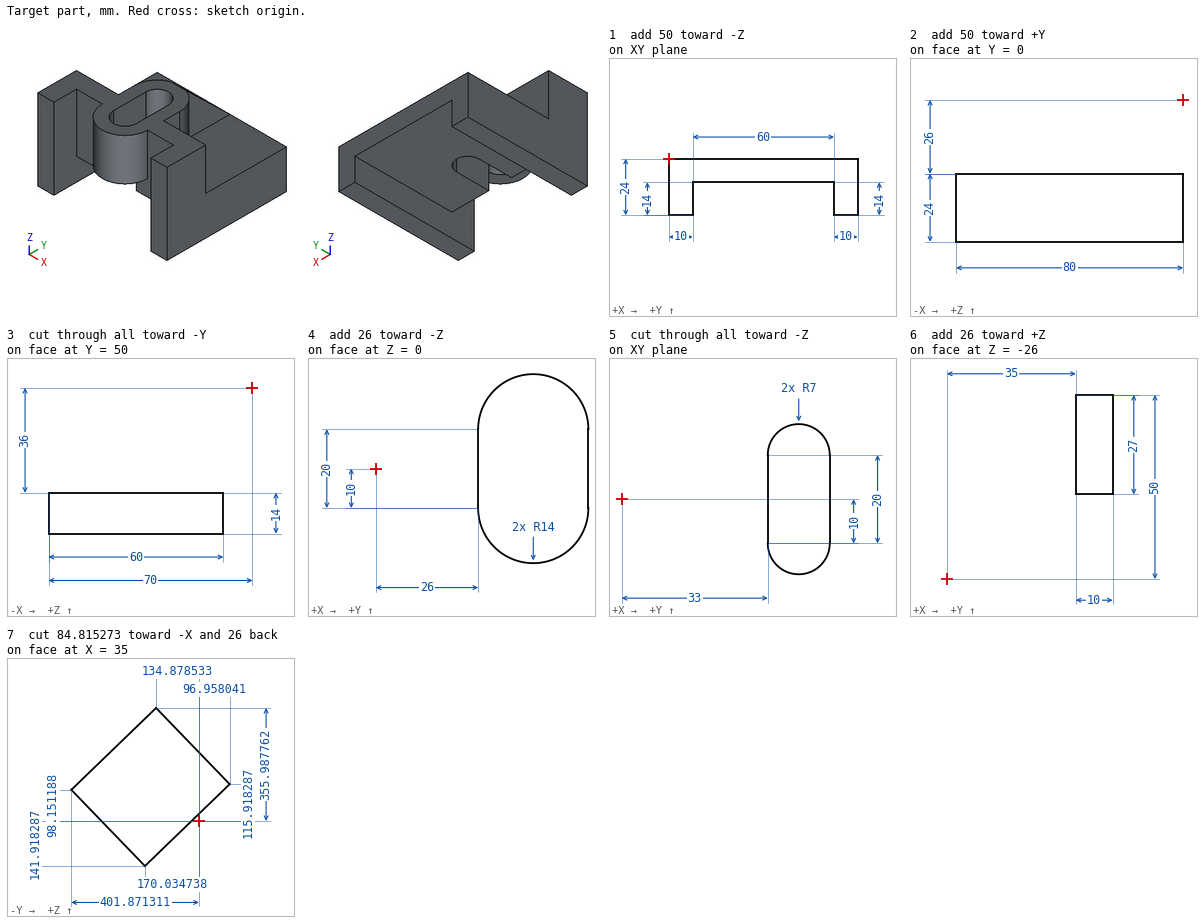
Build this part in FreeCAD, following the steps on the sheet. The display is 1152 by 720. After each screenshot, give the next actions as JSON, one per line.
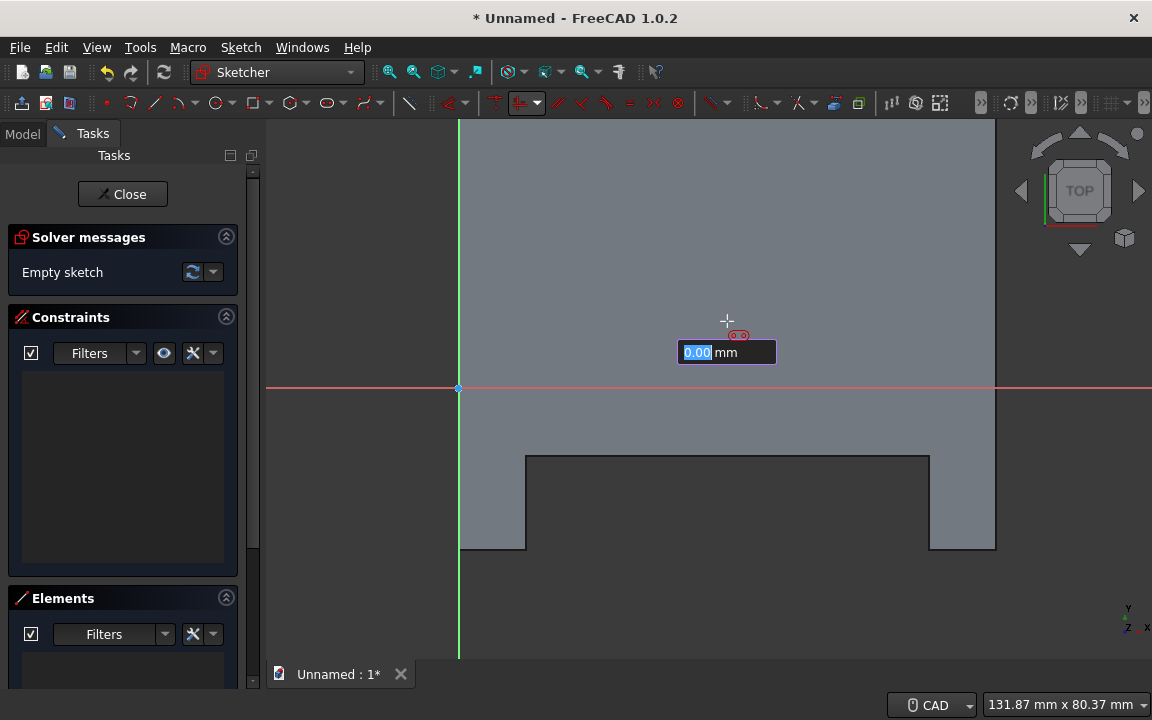
{"action": "left_click", "coordinate": [633, 368]}
{"action": "key", "text": "Escape"}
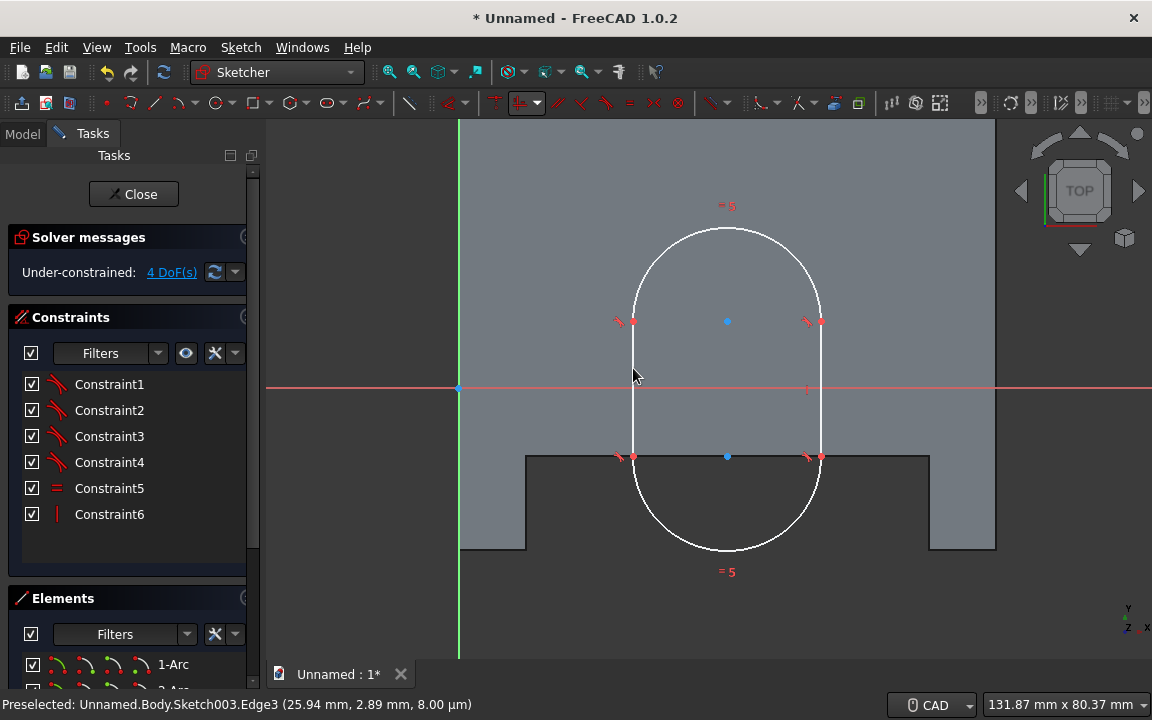
{"action": "left_click", "coordinate": [448, 104]}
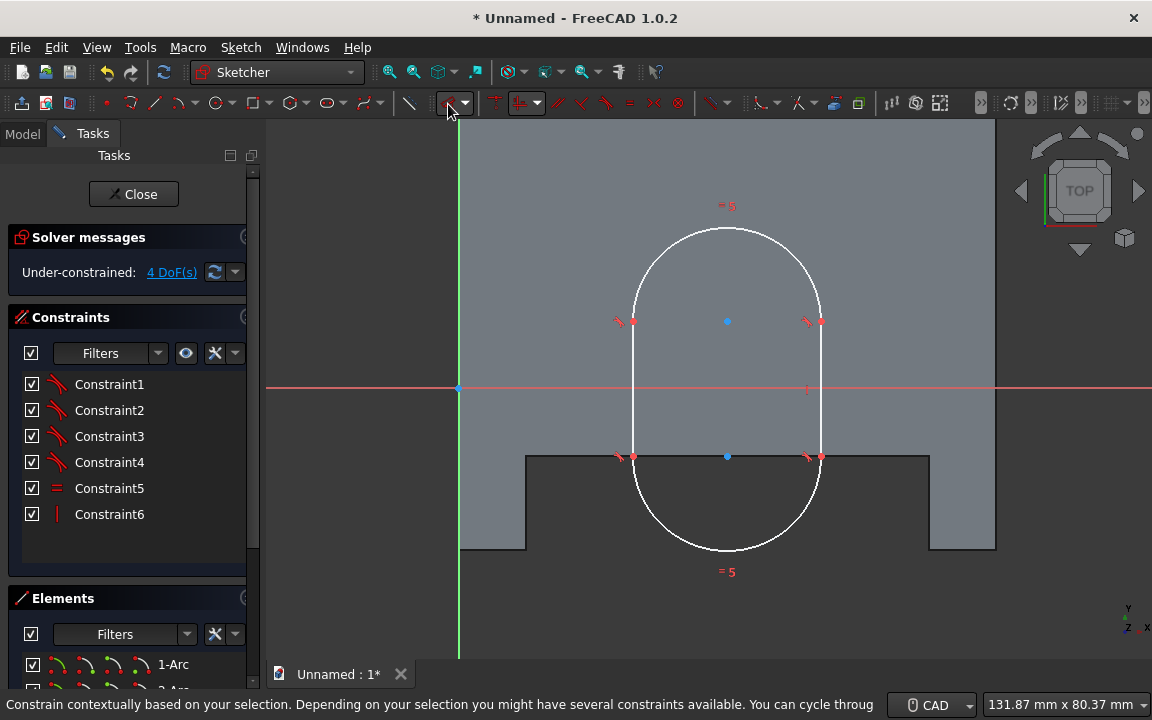
{"action": "left_click", "coordinate": [672, 533]}
{"action": "left_click", "coordinate": [653, 559]}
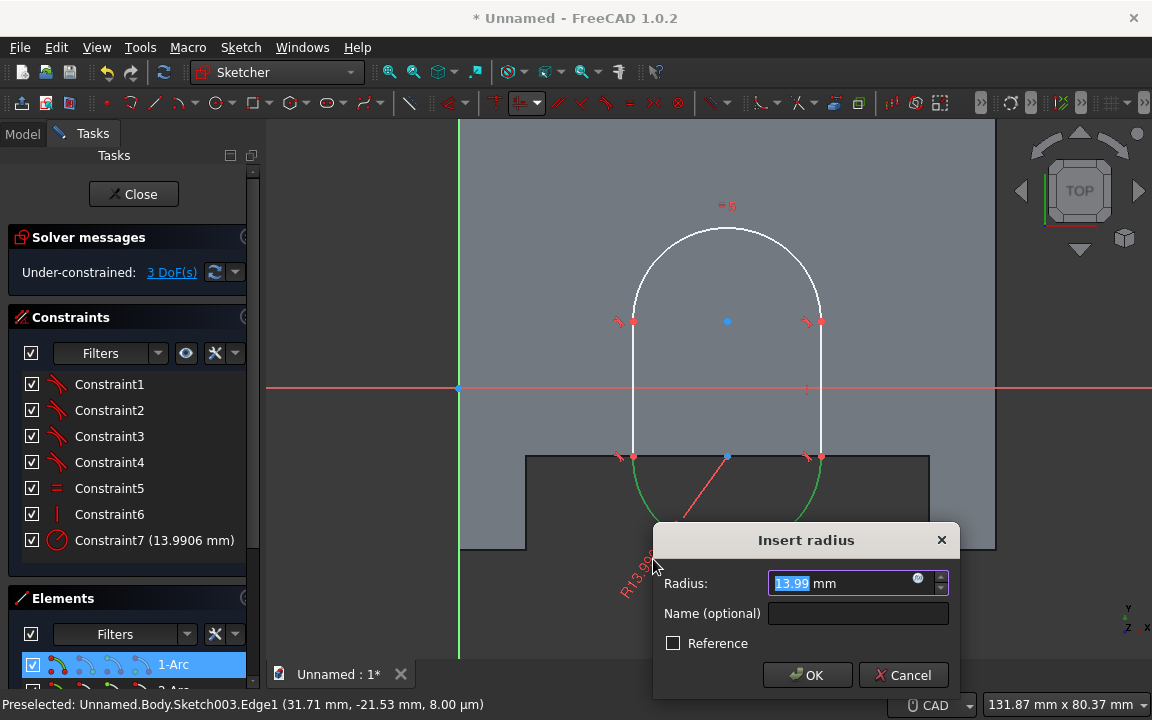
{"action": "type", "text": "14"}
{"action": "key", "text": "Return"}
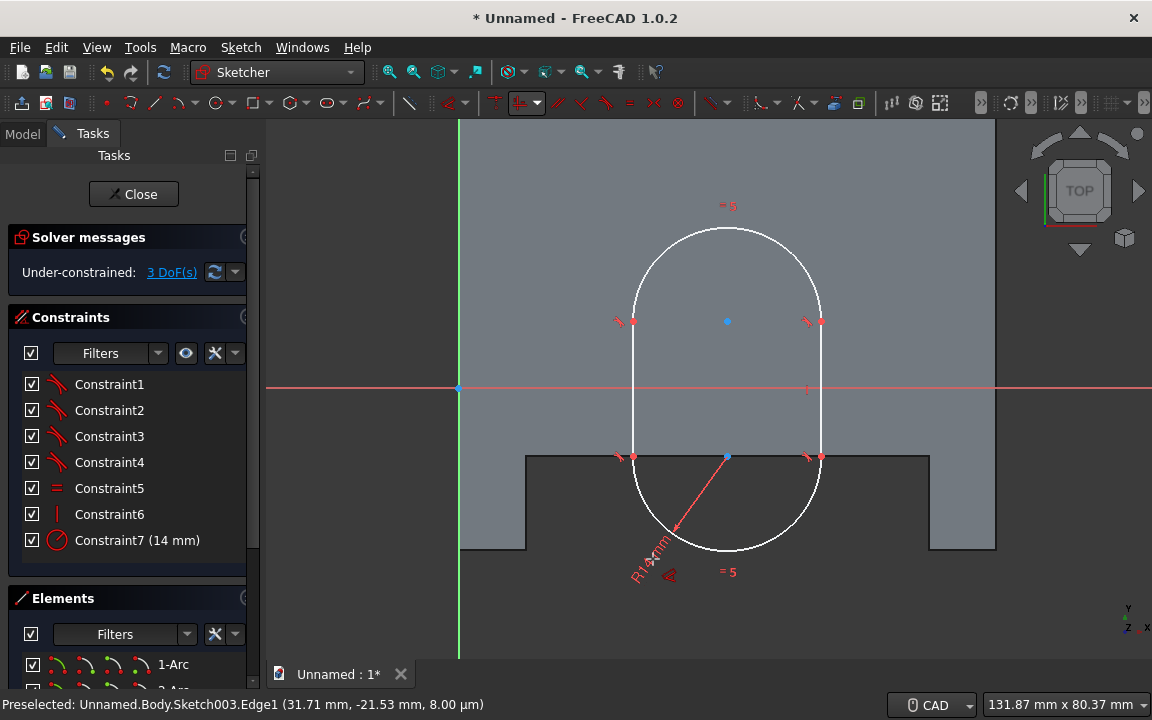
{"action": "left_click", "coordinate": [633, 416]}
{"action": "left_click", "coordinate": [599, 358]}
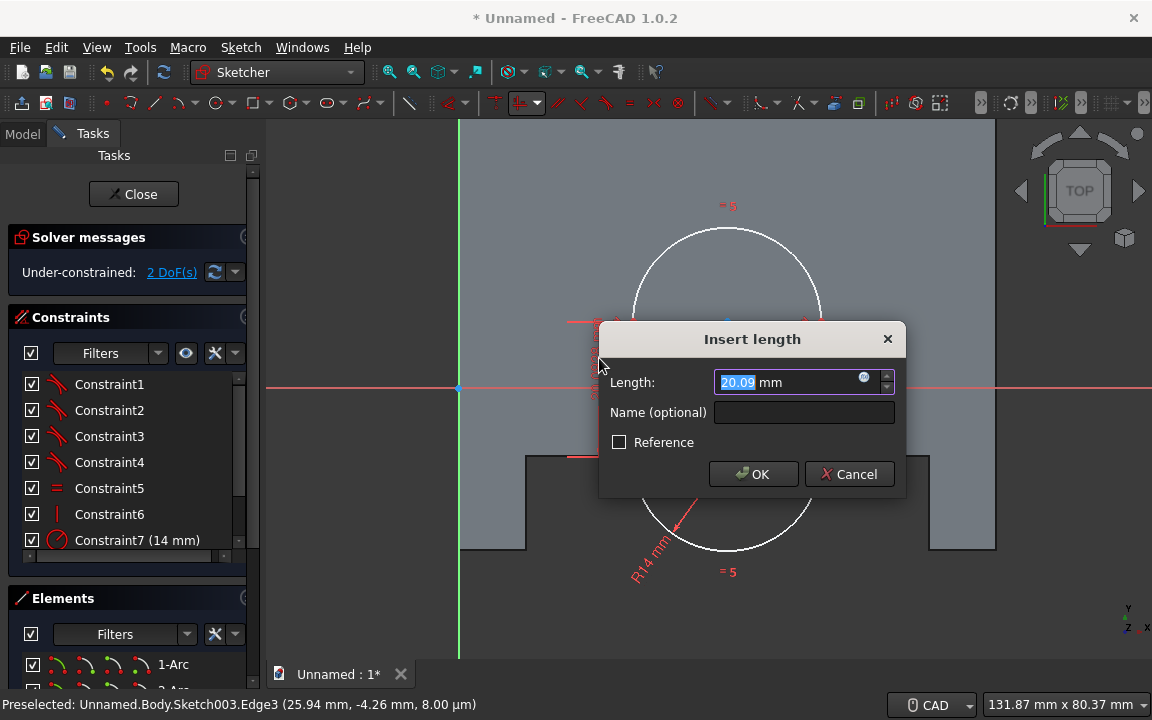
{"action": "type", "text": "20"}
{"action": "key", "text": "Return"}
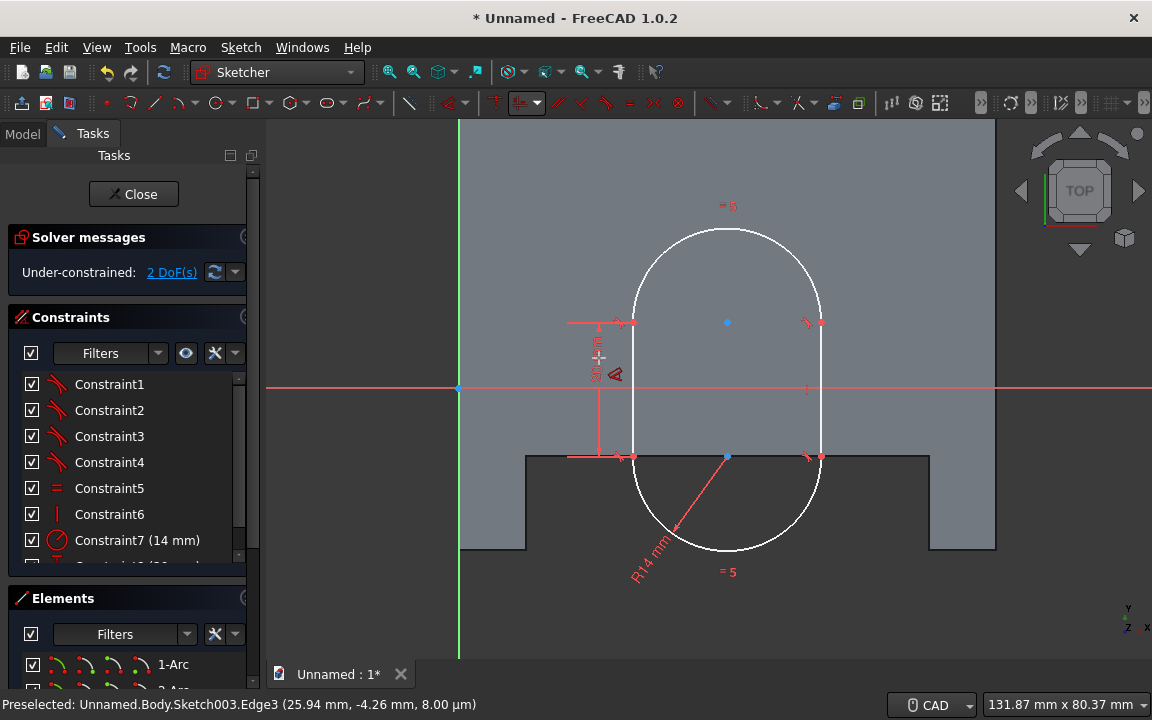
{"action": "left_click", "coordinate": [633, 457]}
{"action": "left_click", "coordinate": [546, 491]}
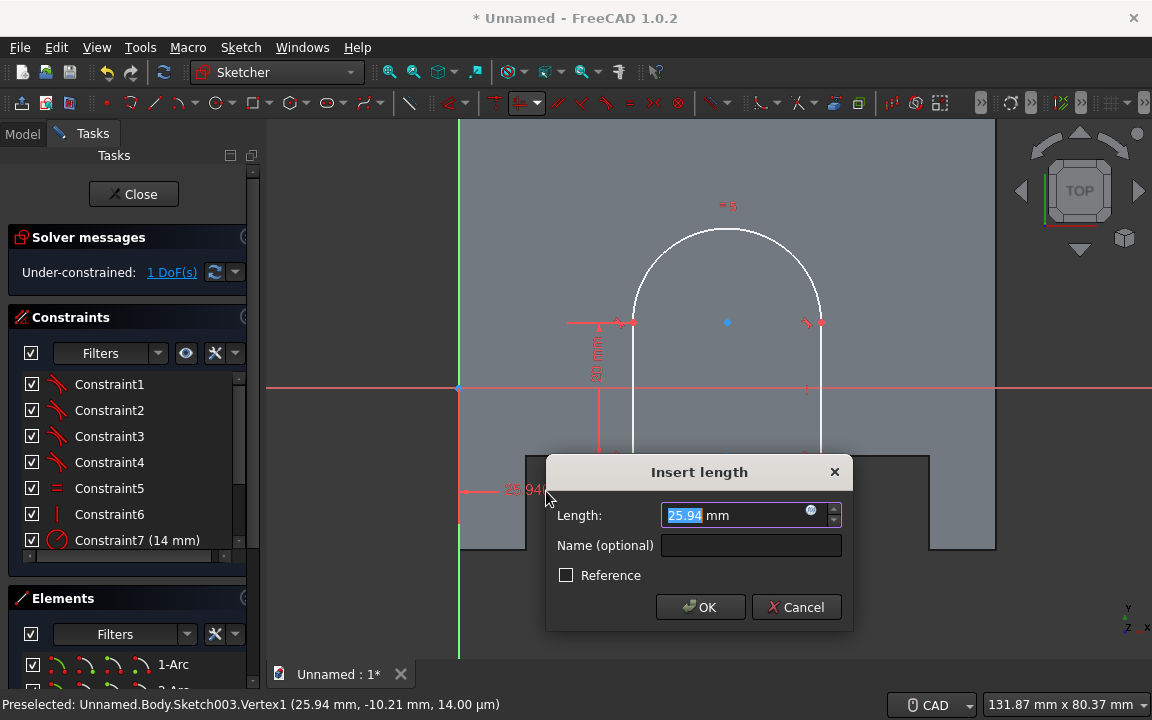
{"action": "type", "text": "26"}
{"action": "key", "text": "Return"}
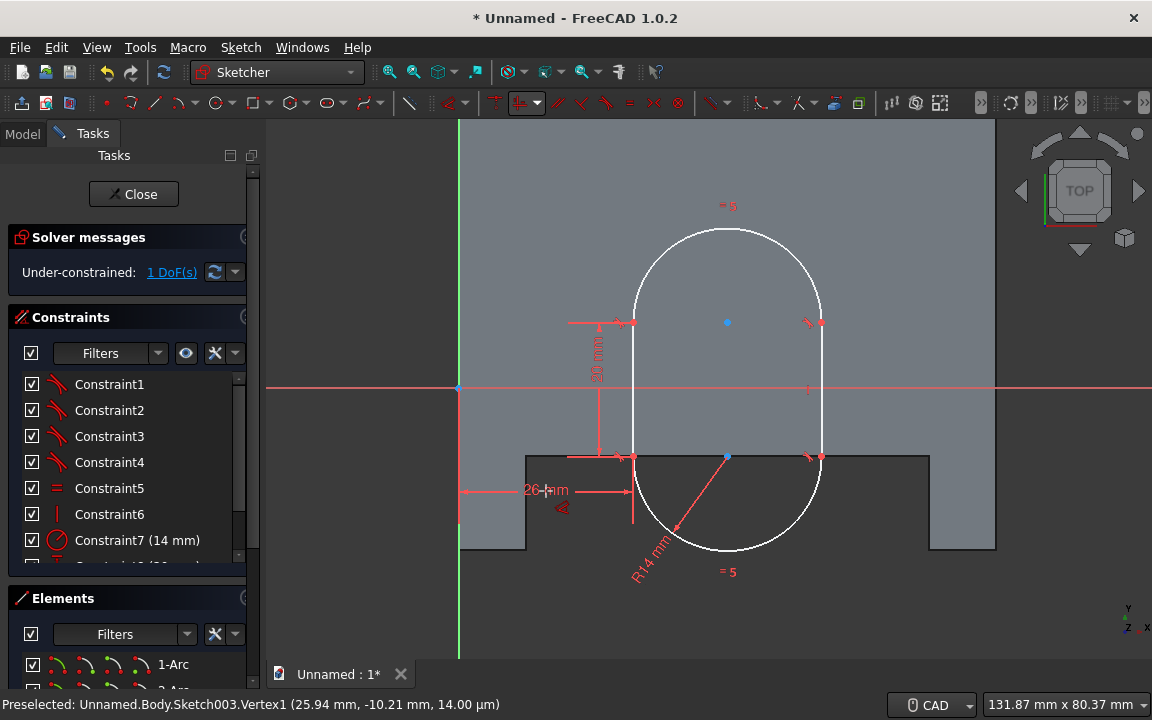
{"action": "left_click", "coordinate": [633, 457]}
{"action": "left_click", "coordinate": [425, 423]}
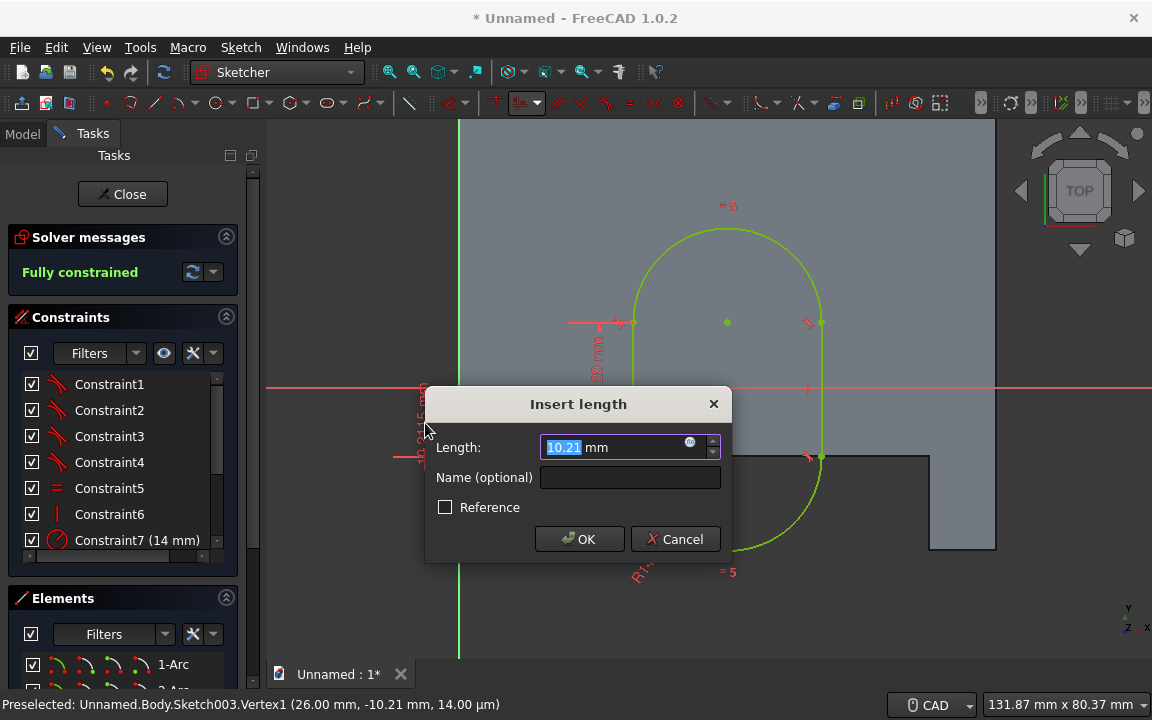
{"action": "type", "text": "10"}
{"action": "key", "text": "Return"}
{"action": "key", "text": "Escape"}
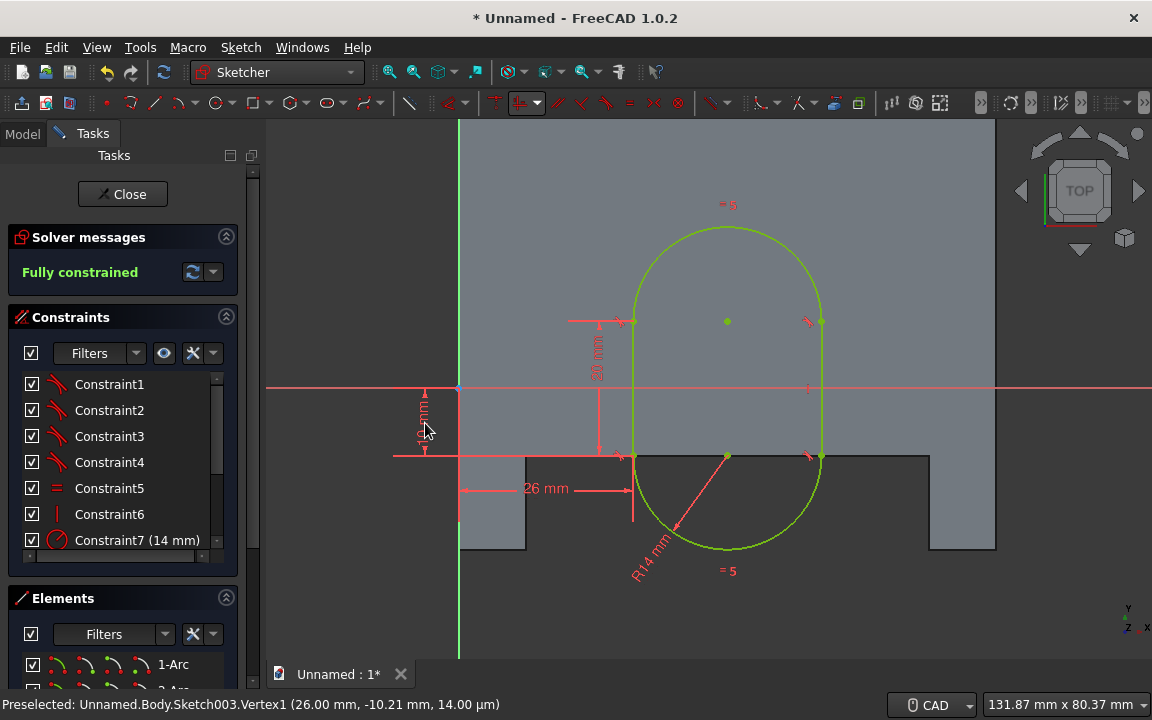
{"action": "left_click", "coordinate": [123, 194]}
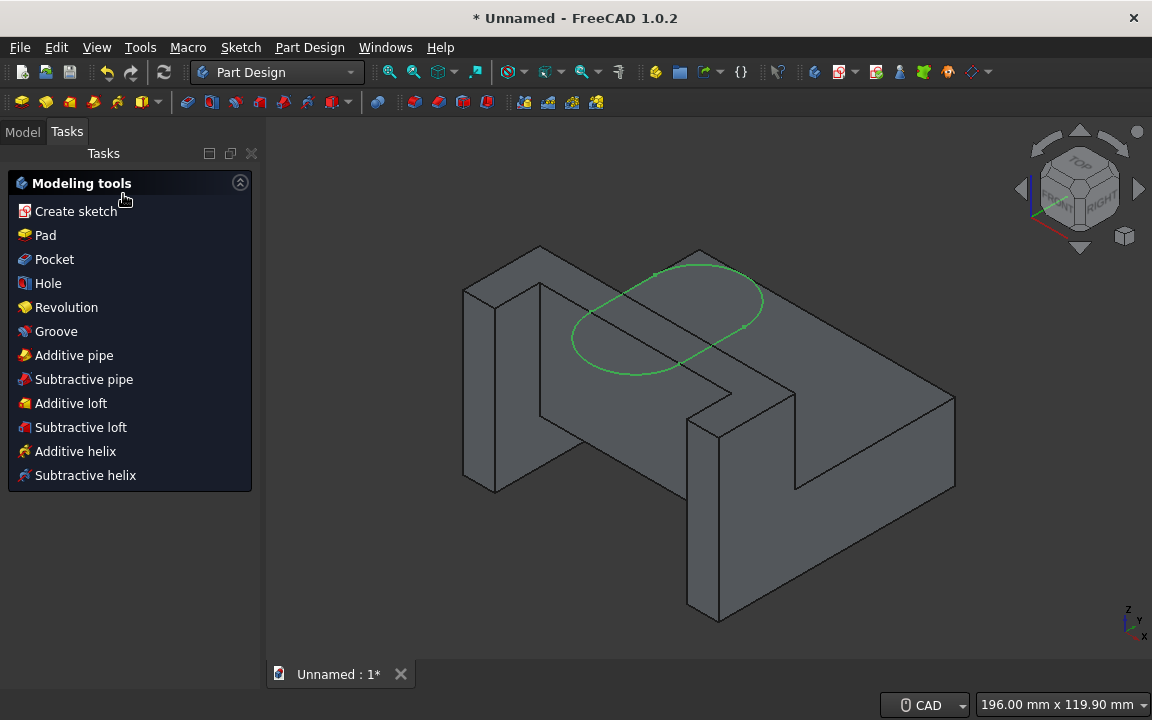
{"action": "left_click", "coordinate": [22, 102]}